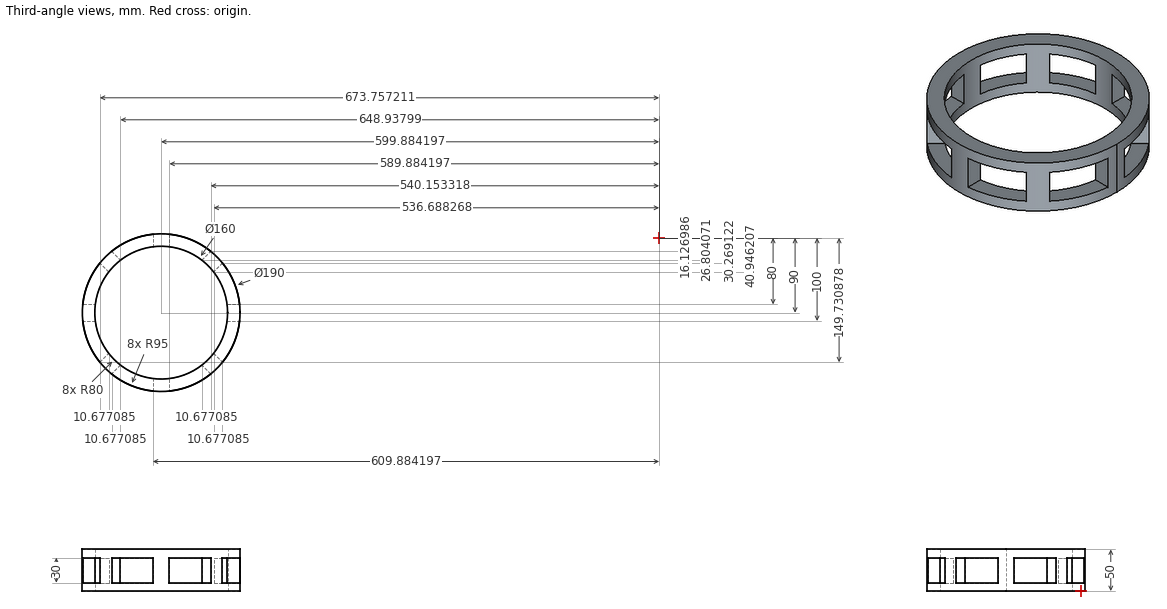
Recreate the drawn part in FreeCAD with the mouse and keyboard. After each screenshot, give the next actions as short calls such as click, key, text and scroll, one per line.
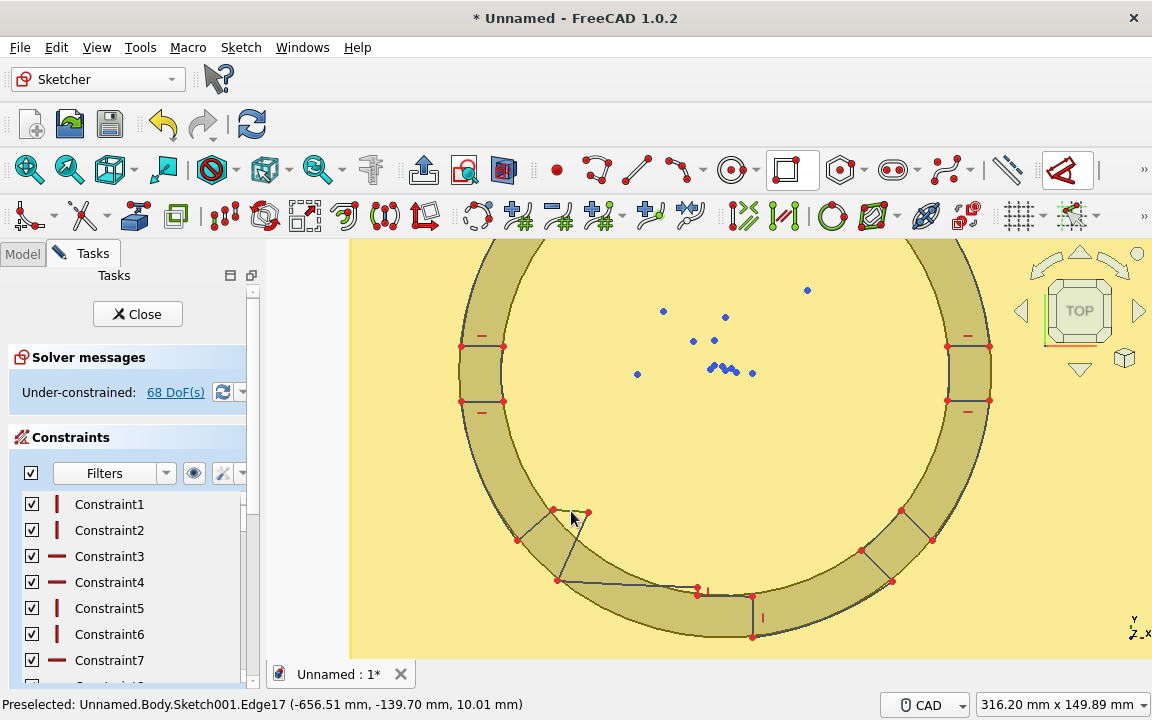
click(797, 628)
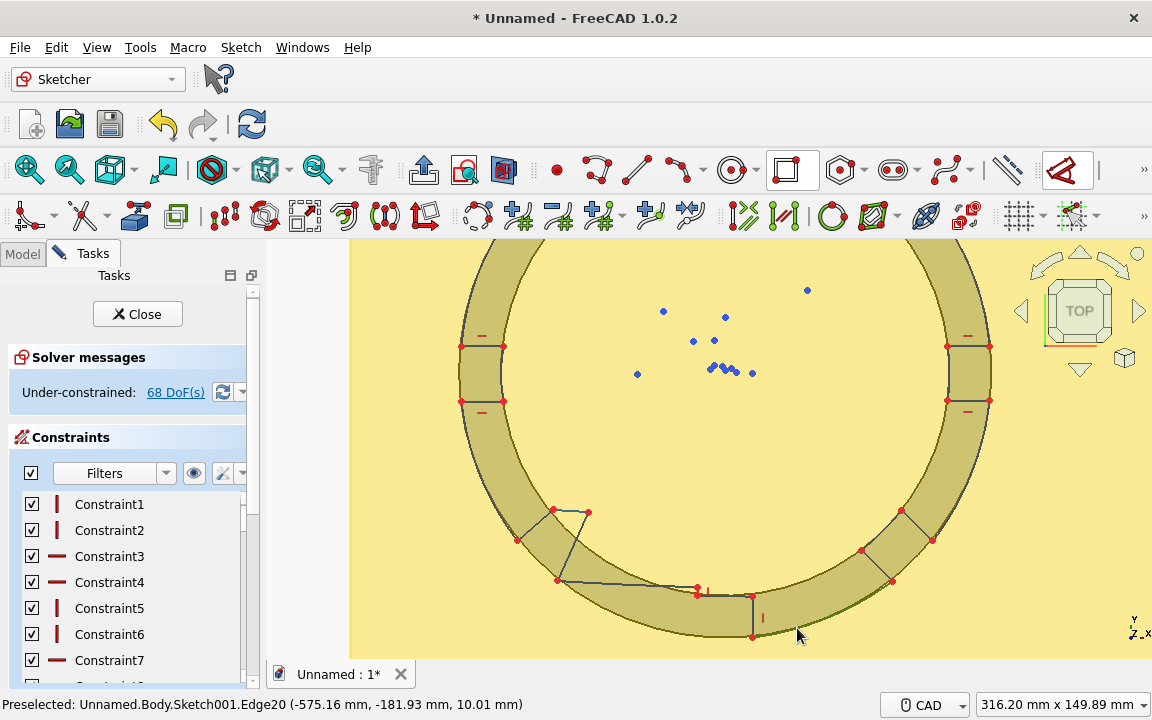
key(c)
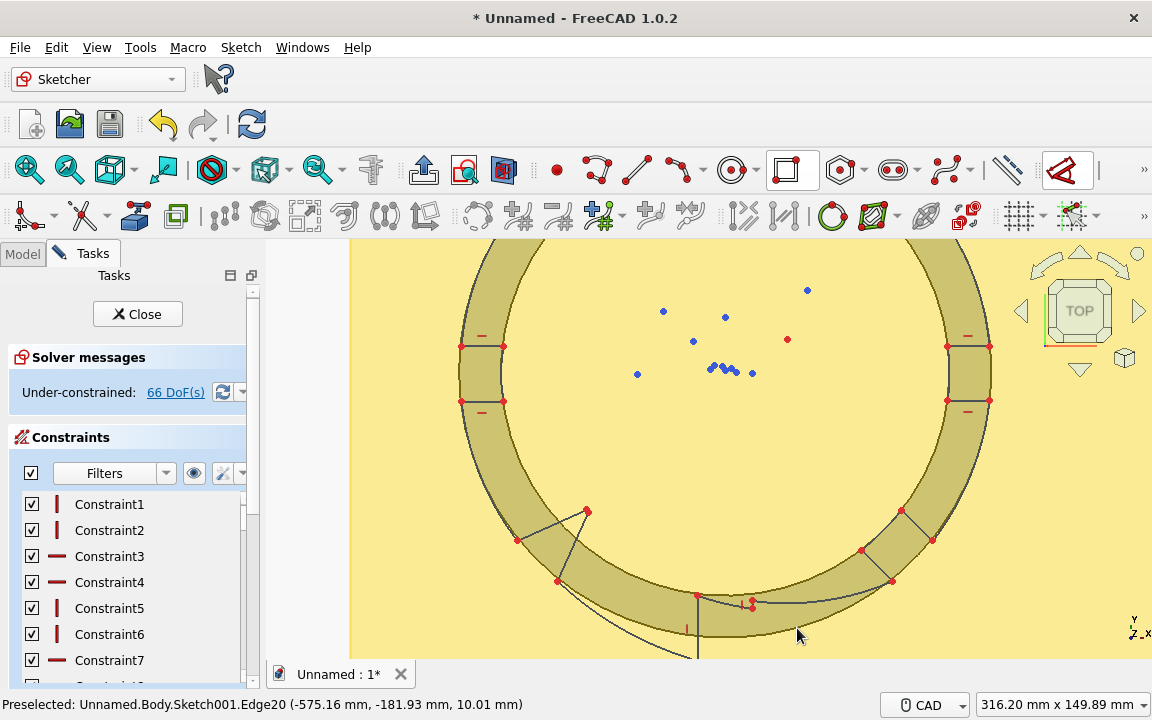
scroll(588, 511, up, 11)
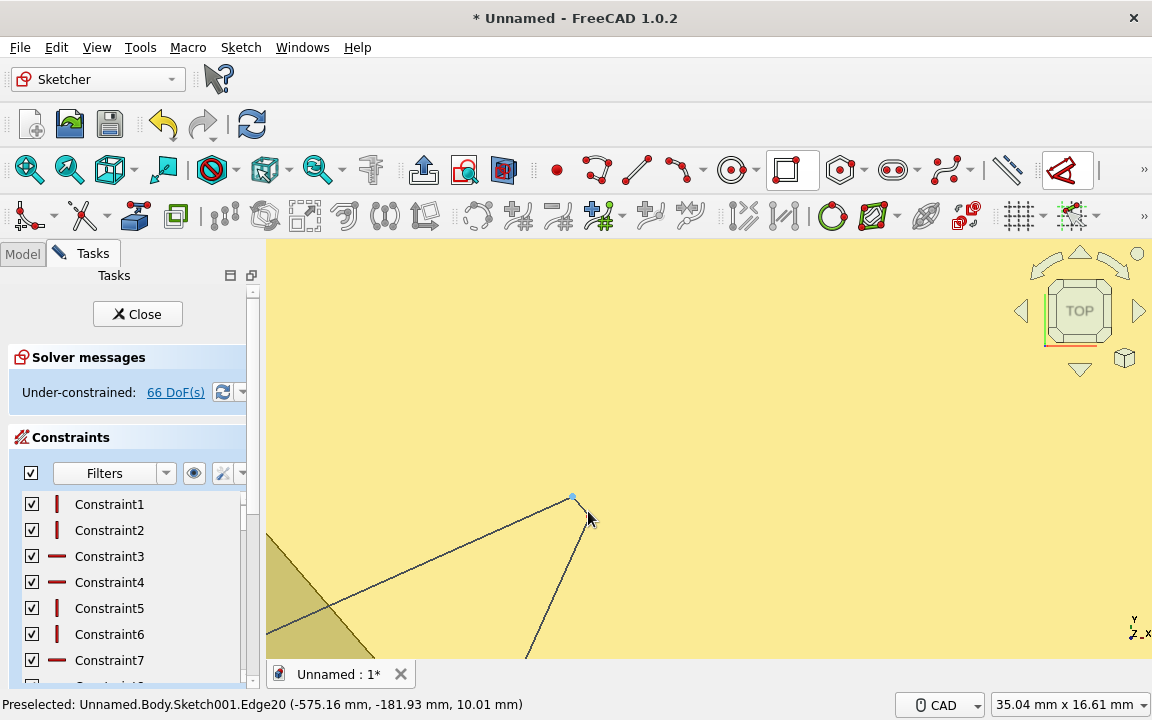
click(581, 507)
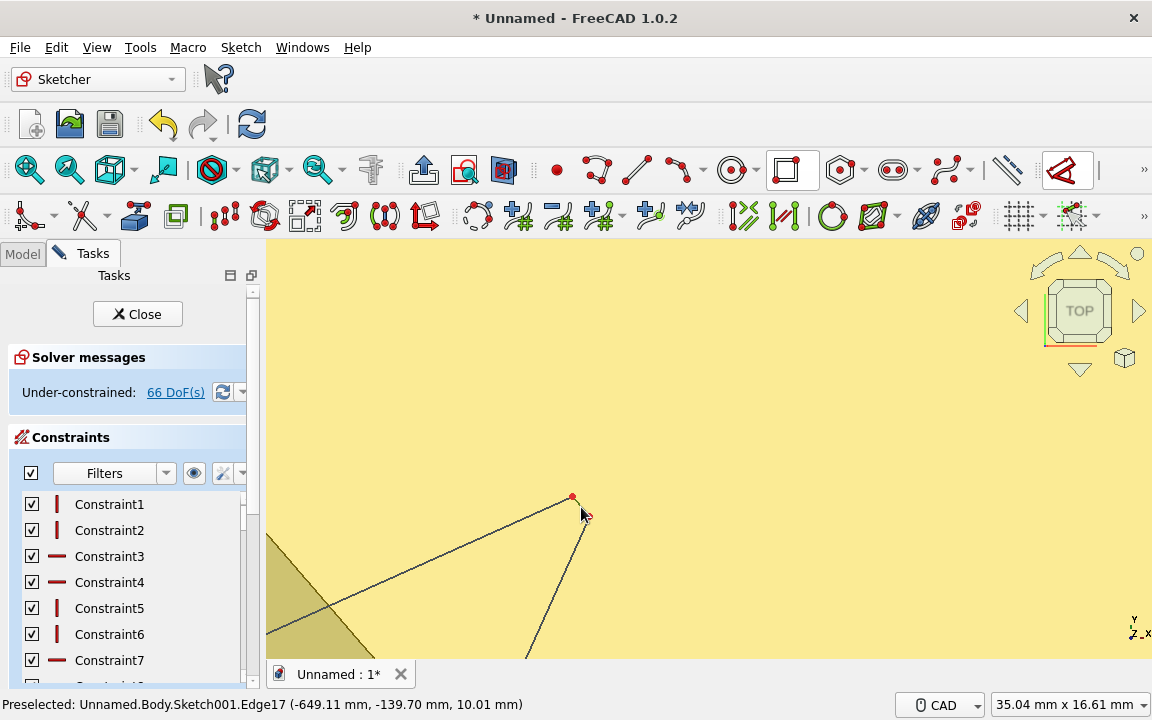
scroll(579, 512, down, 15)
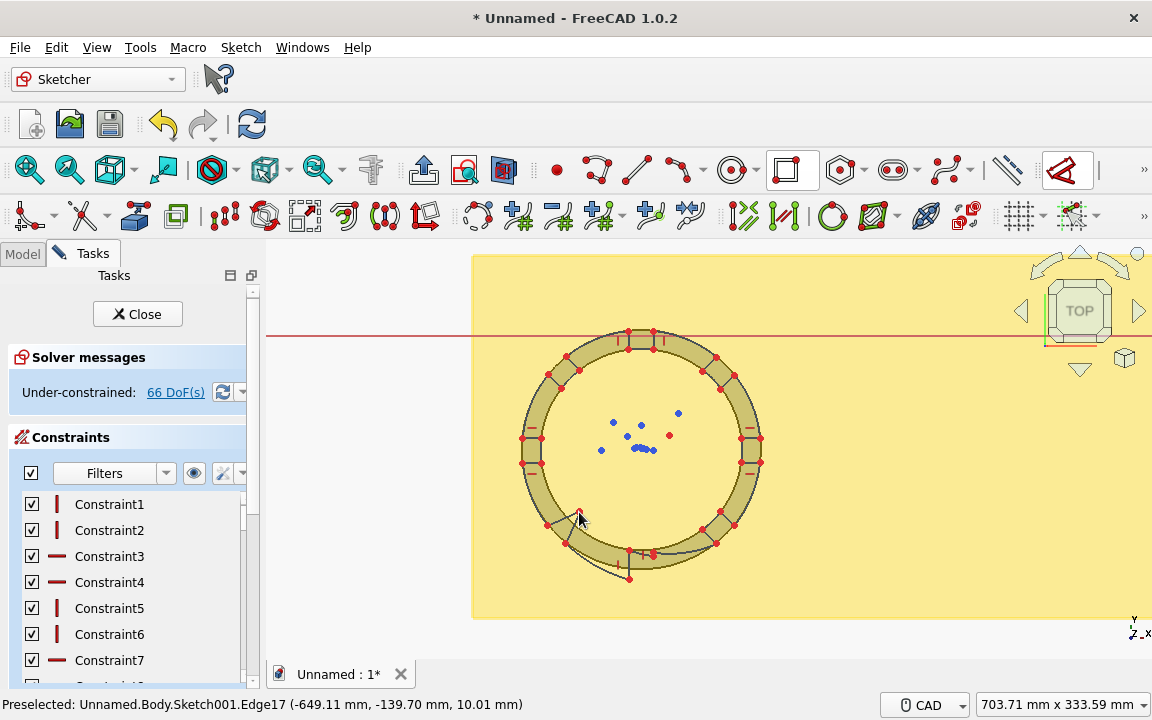
scroll(708, 525, up, 3)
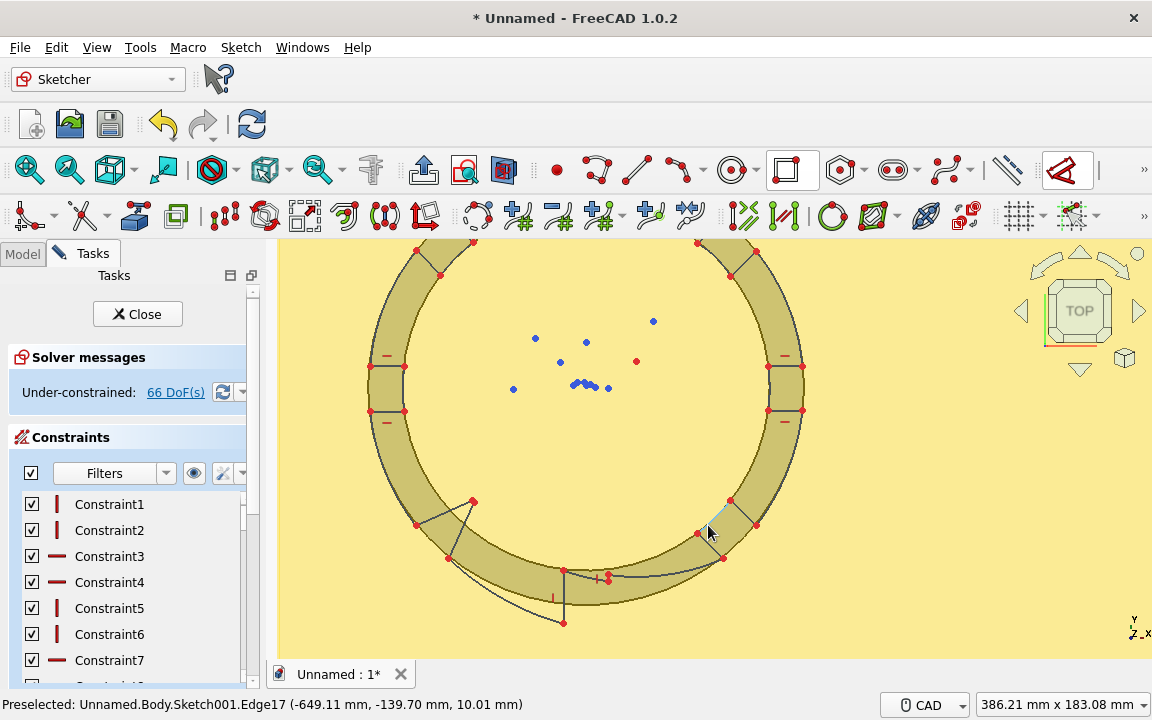
click(708, 524)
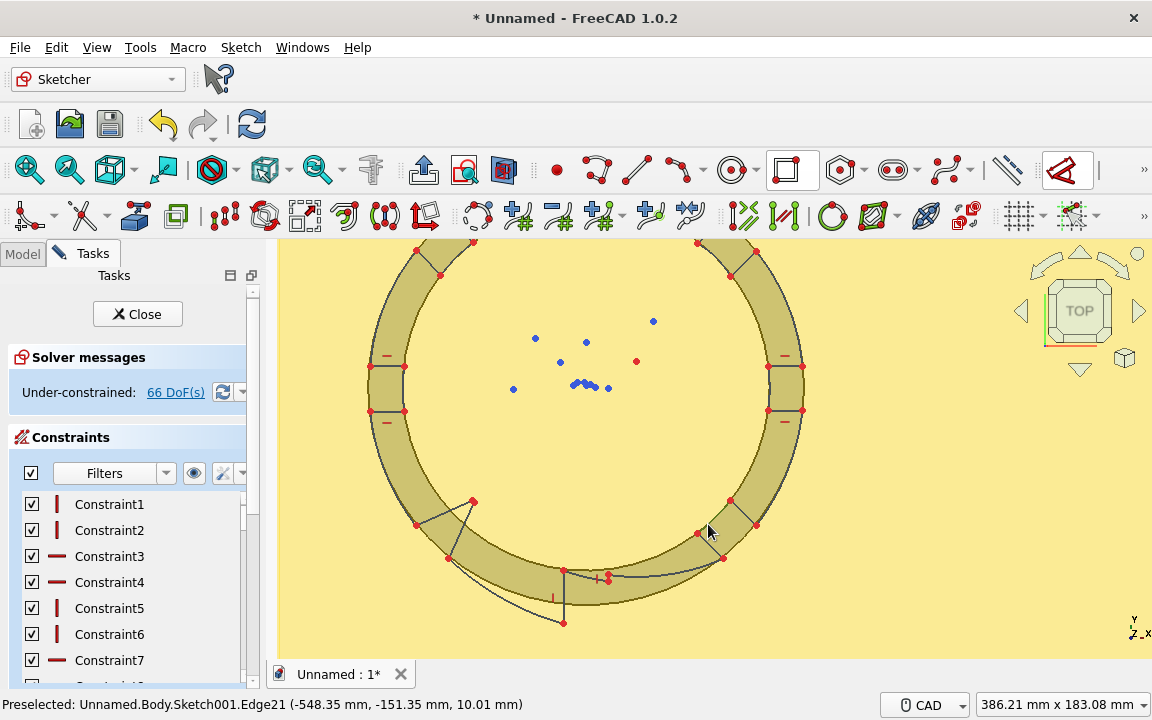
key(c)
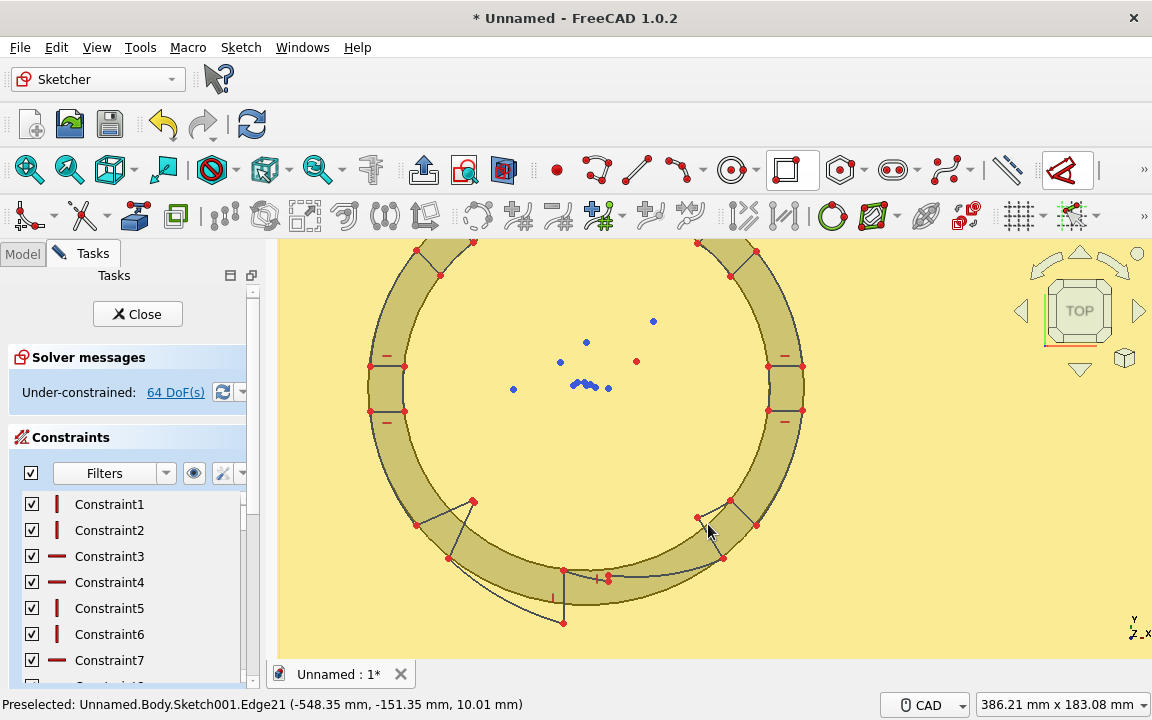
scroll(473, 501, up, 12)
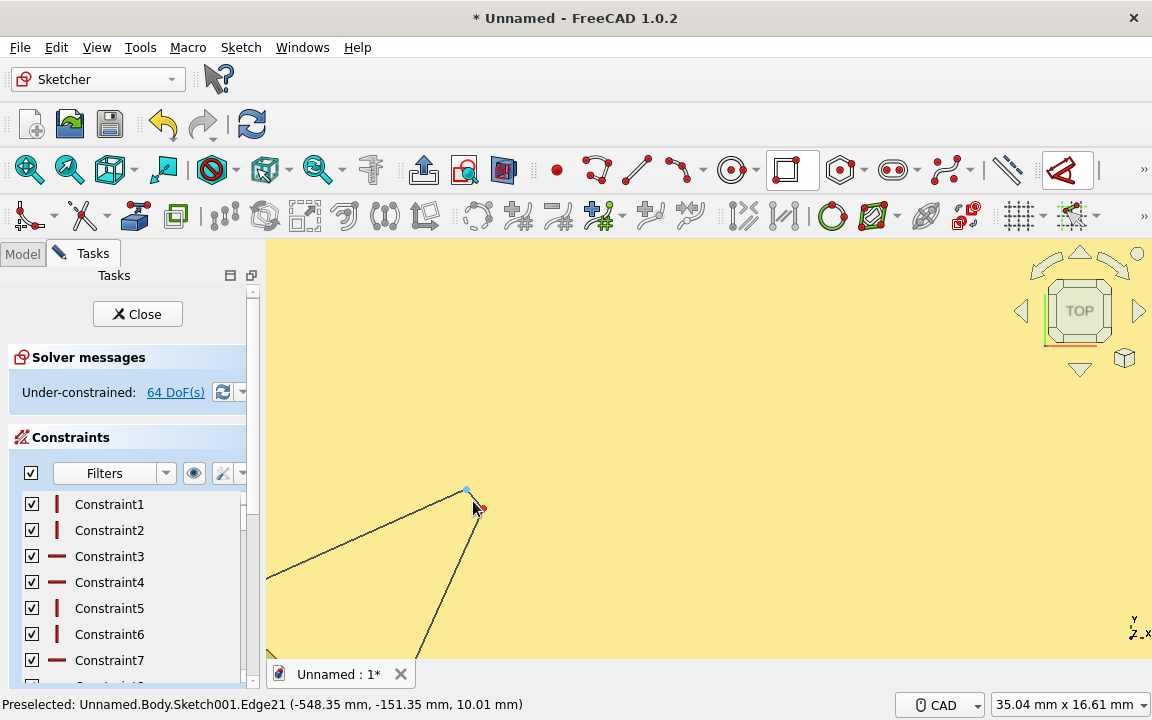
click(475, 499)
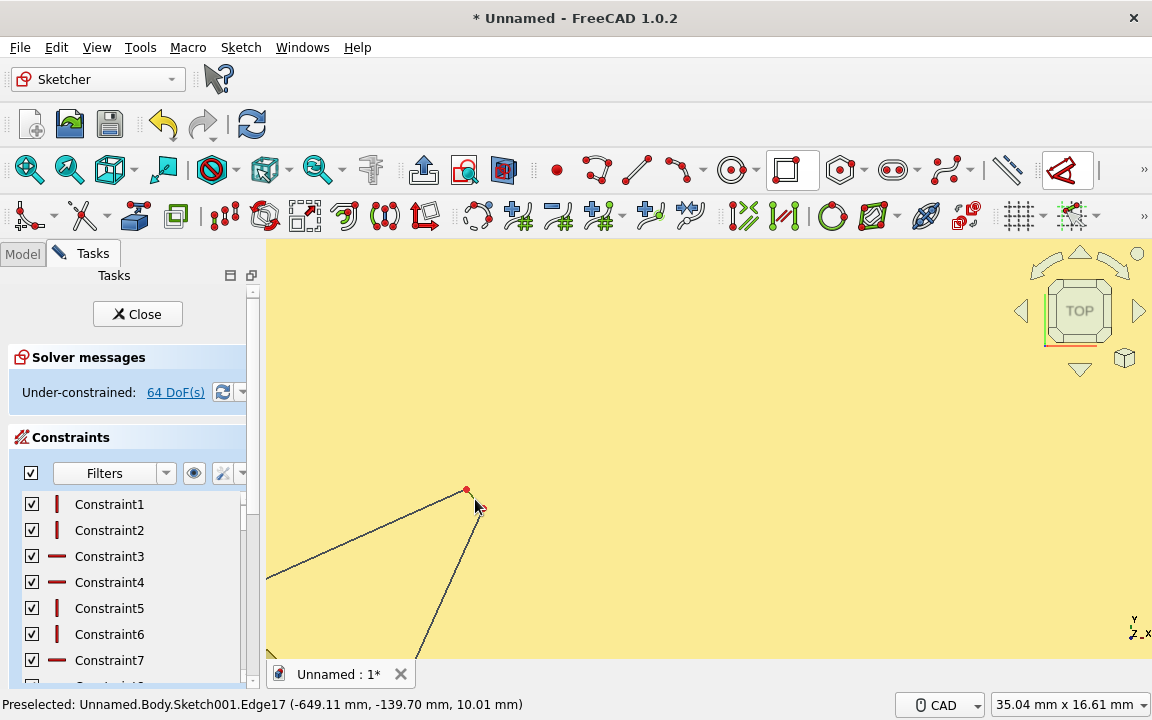
scroll(584, 512, down, 15)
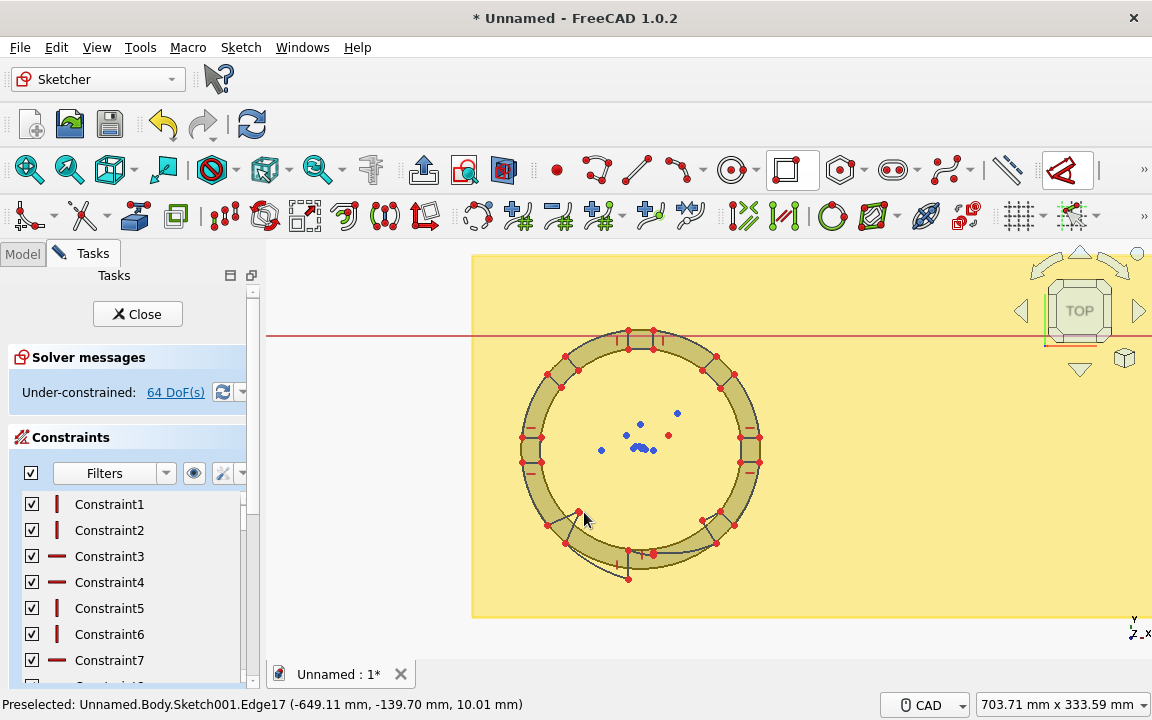
click(745, 508)